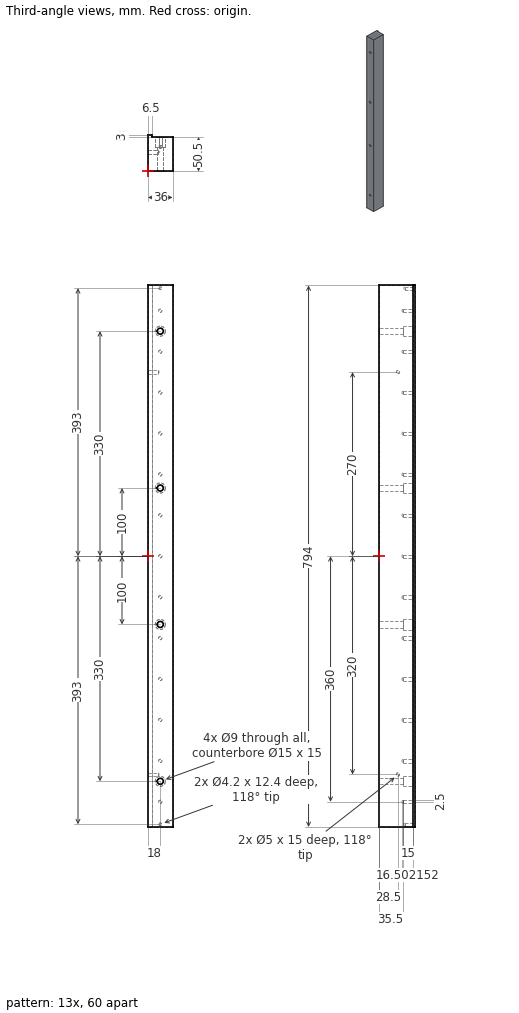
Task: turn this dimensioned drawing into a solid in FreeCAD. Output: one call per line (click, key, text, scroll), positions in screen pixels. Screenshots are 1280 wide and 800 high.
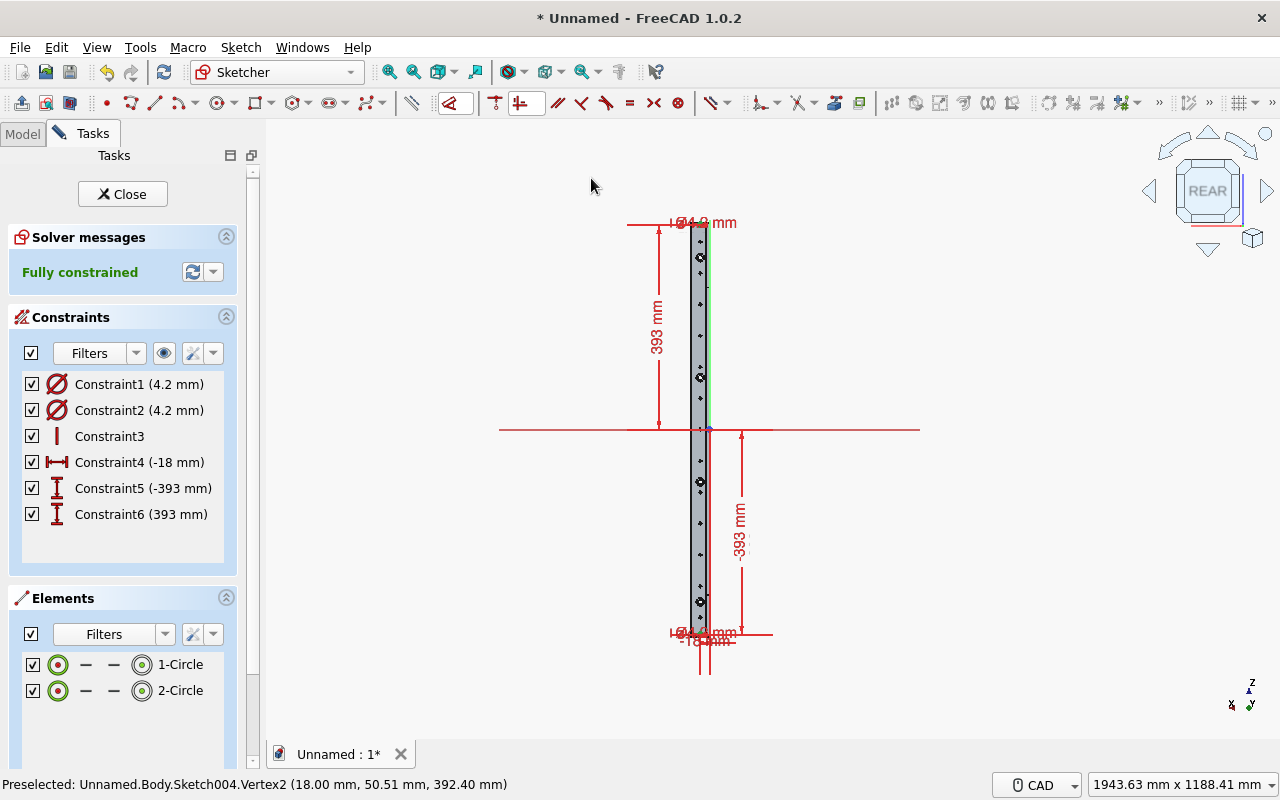
click(123, 194)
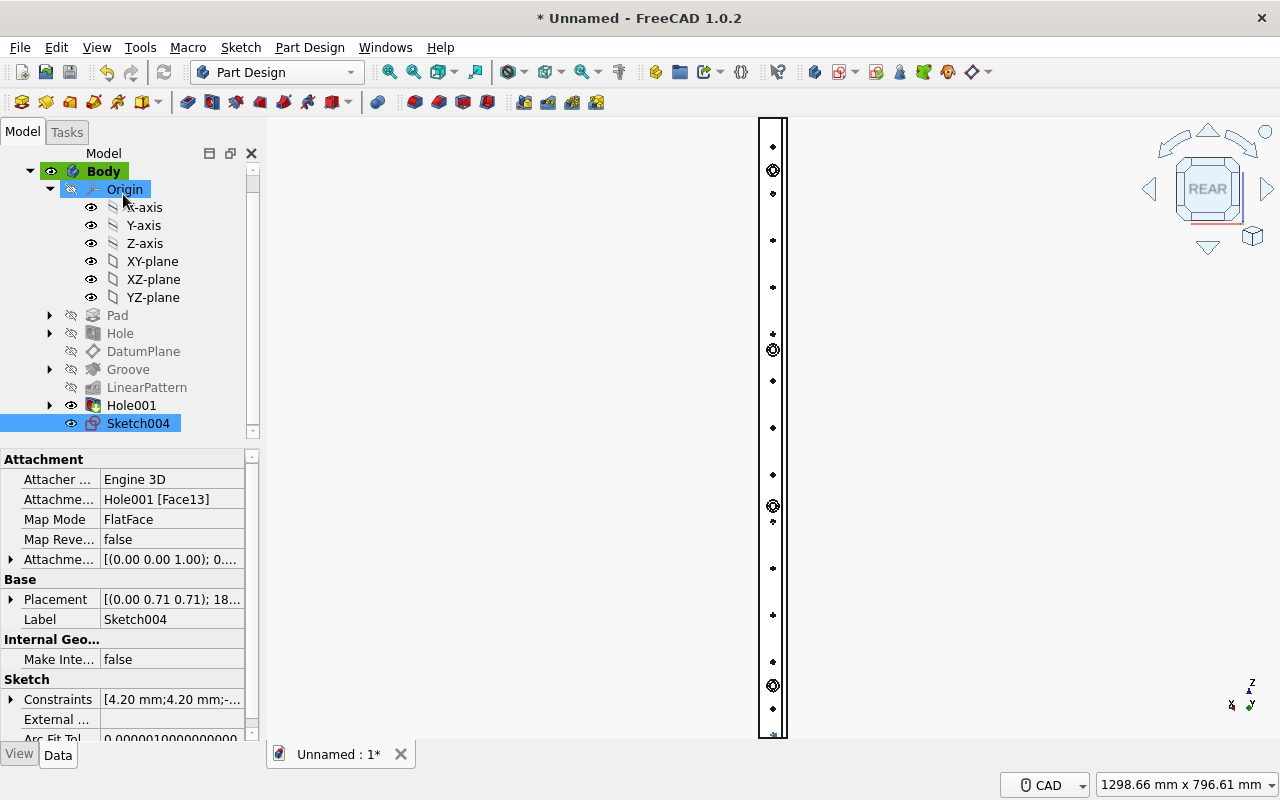
click(212, 102)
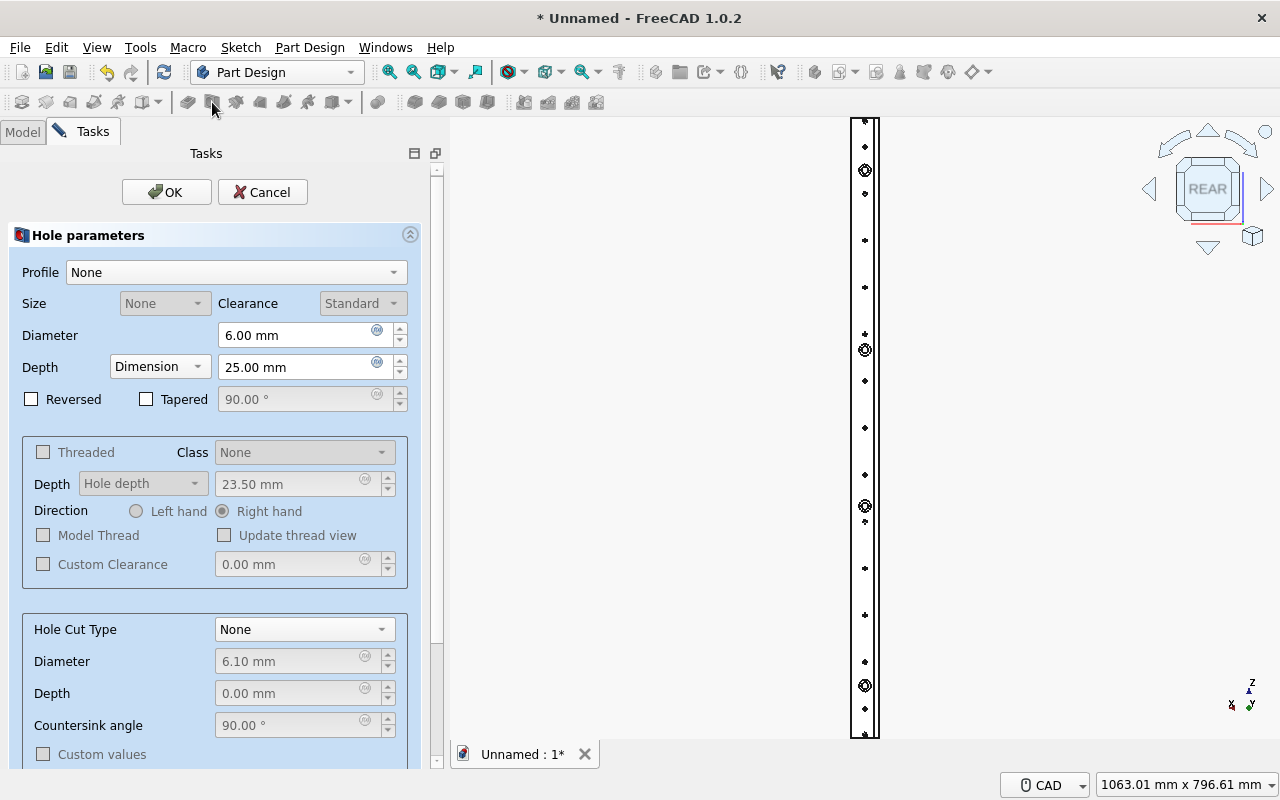
triple_click(305, 335)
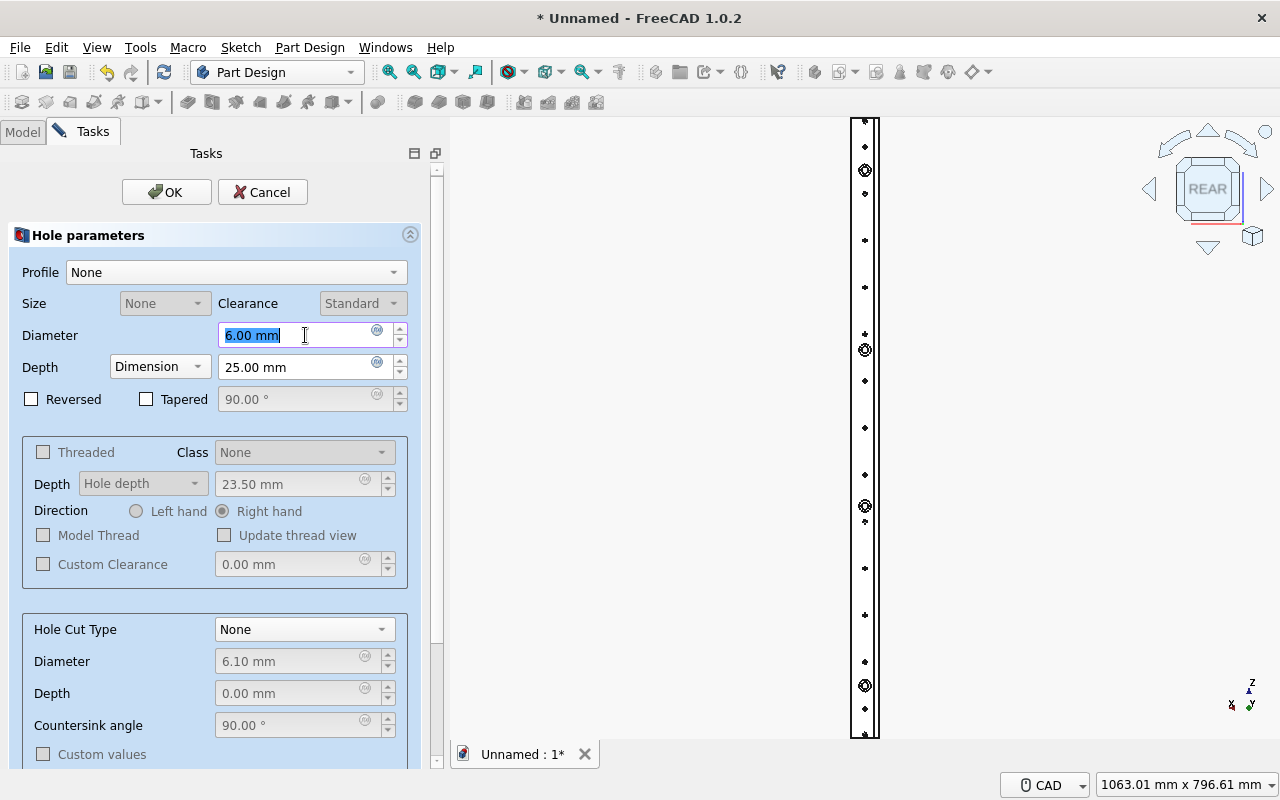
text(4.2)
key(Tab)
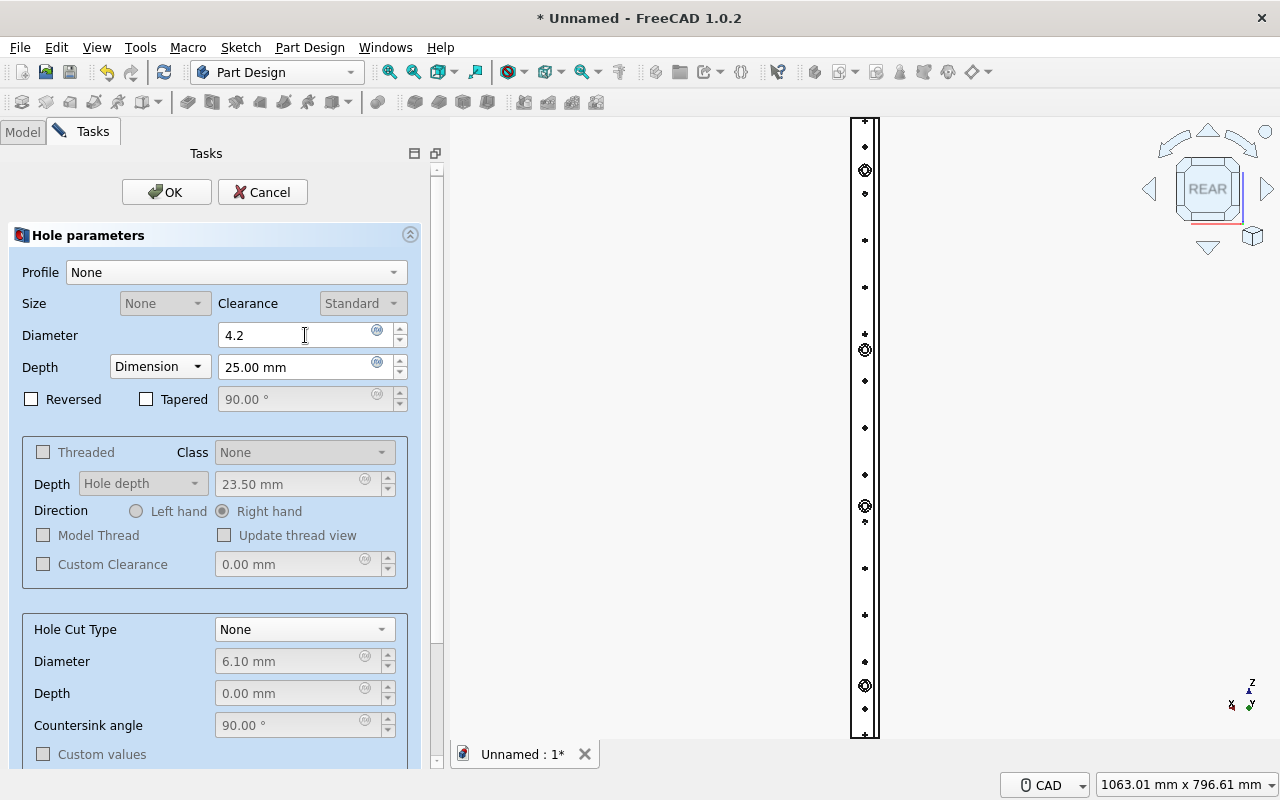
triple_click(305, 367)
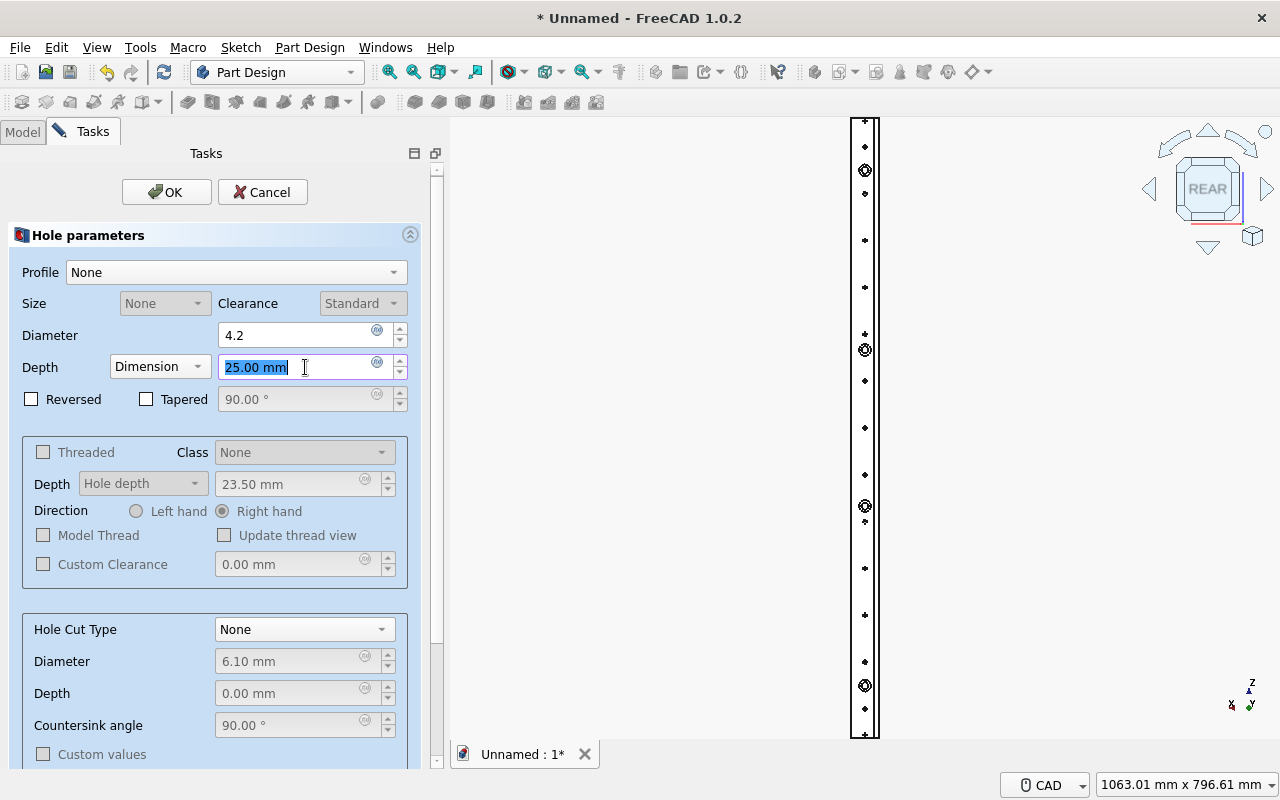
text(12.4)
key(Tab)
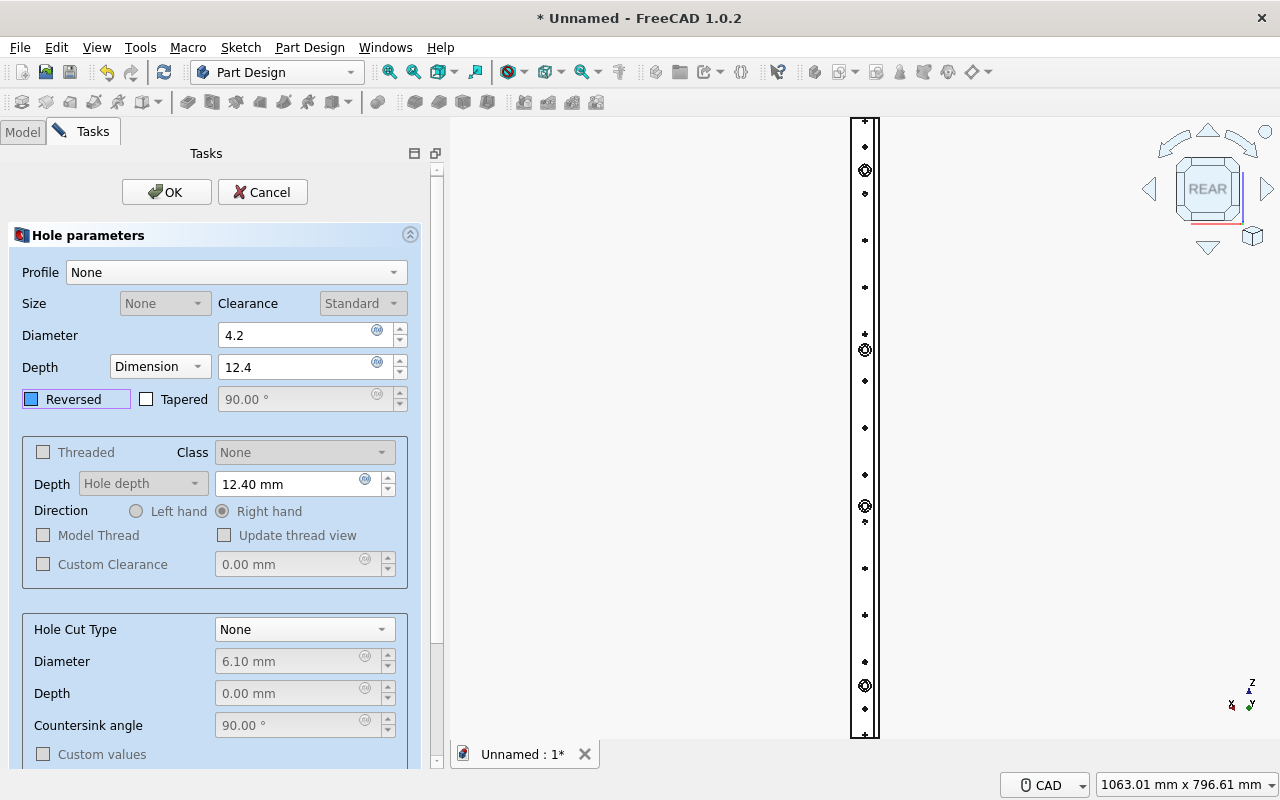
click(167, 192)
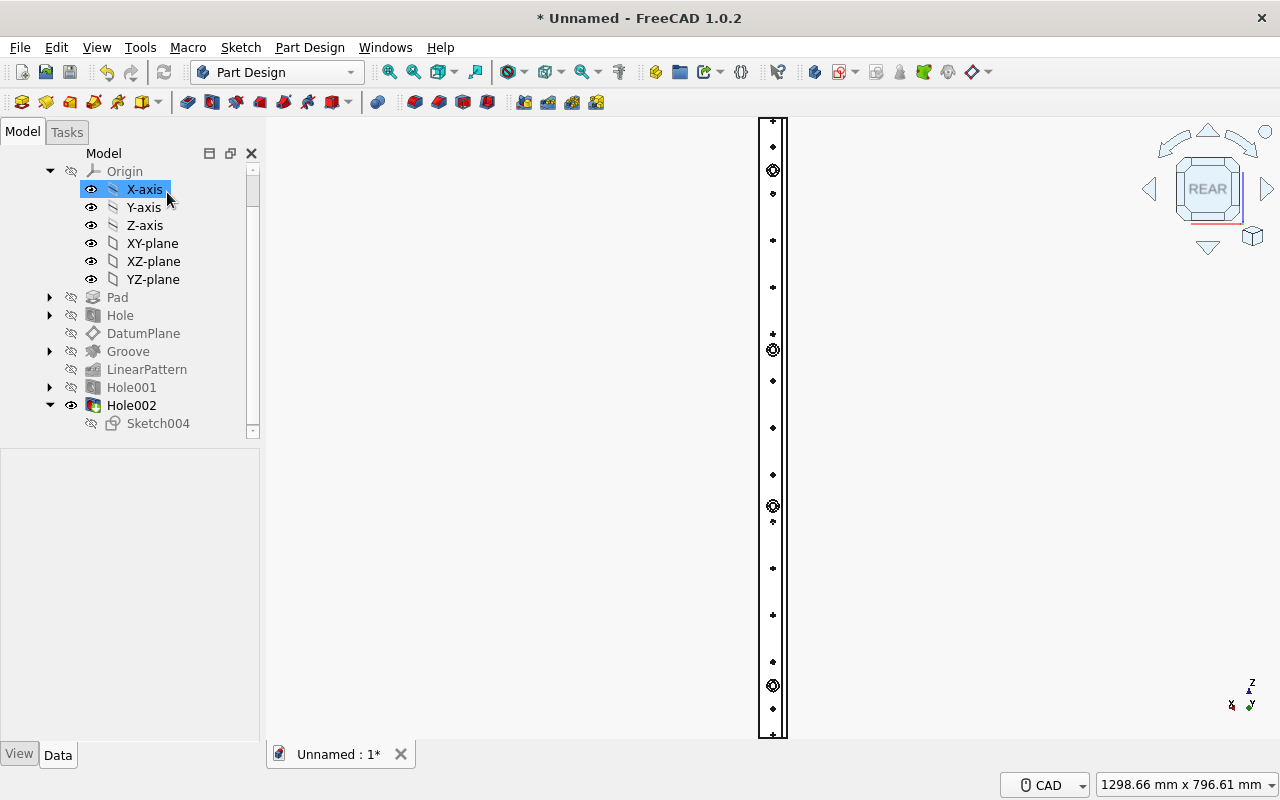
key(0)